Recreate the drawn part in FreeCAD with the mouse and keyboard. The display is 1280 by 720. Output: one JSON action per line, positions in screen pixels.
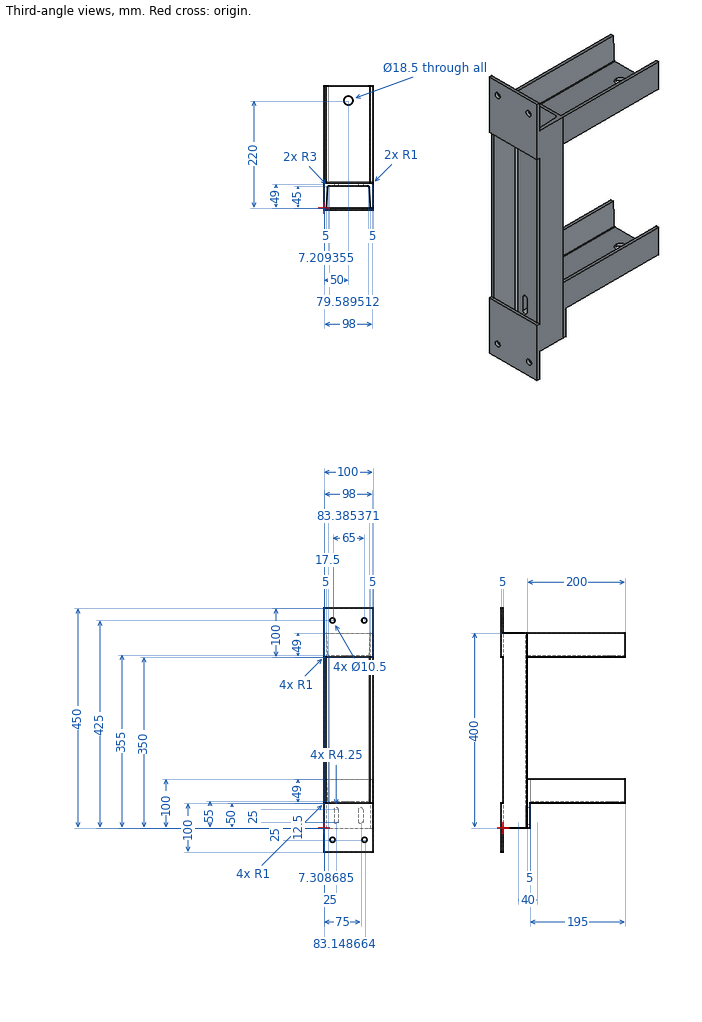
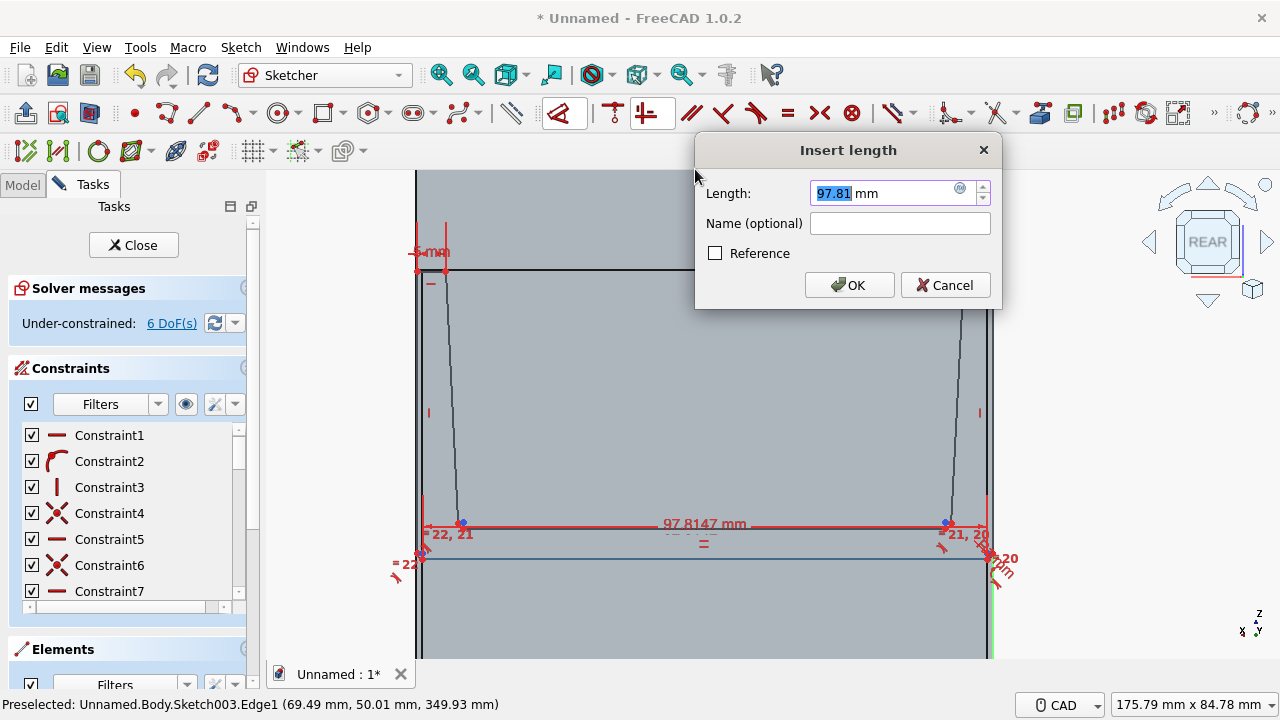
{"action": "type", "text": "98"}
{"action": "key", "text": "Return"}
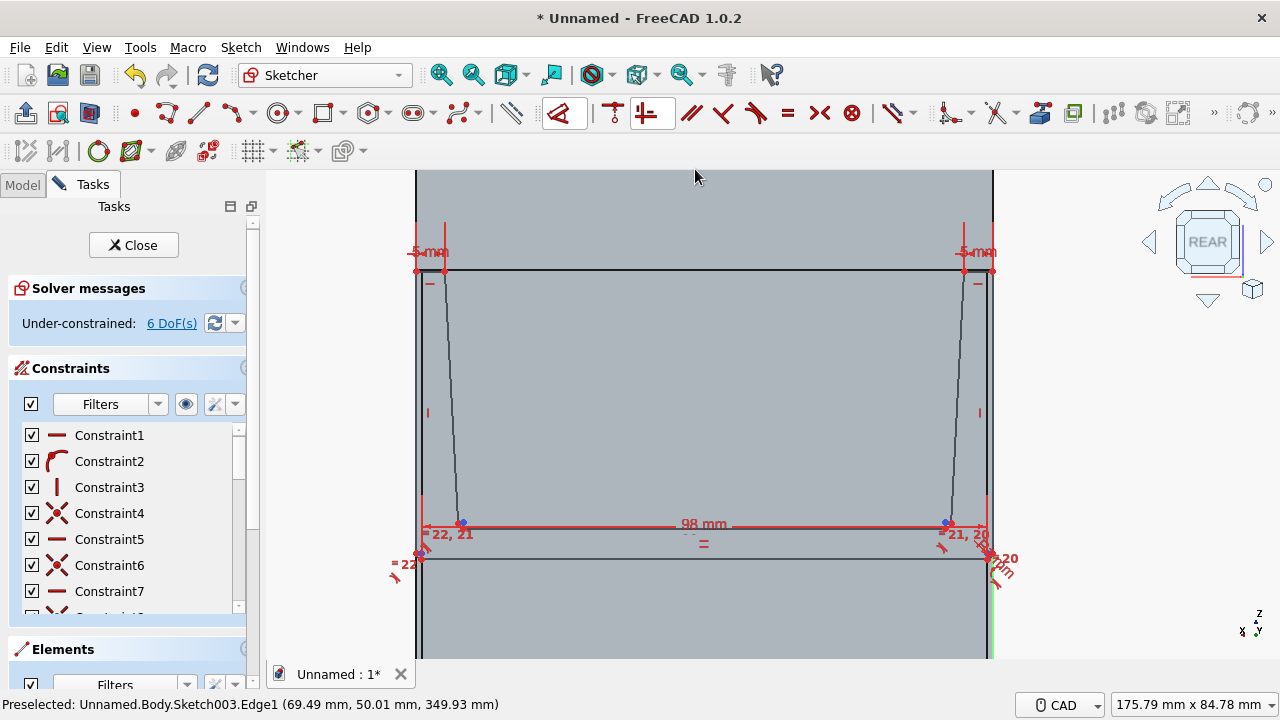
{"action": "left_click", "coordinate": [993, 469]}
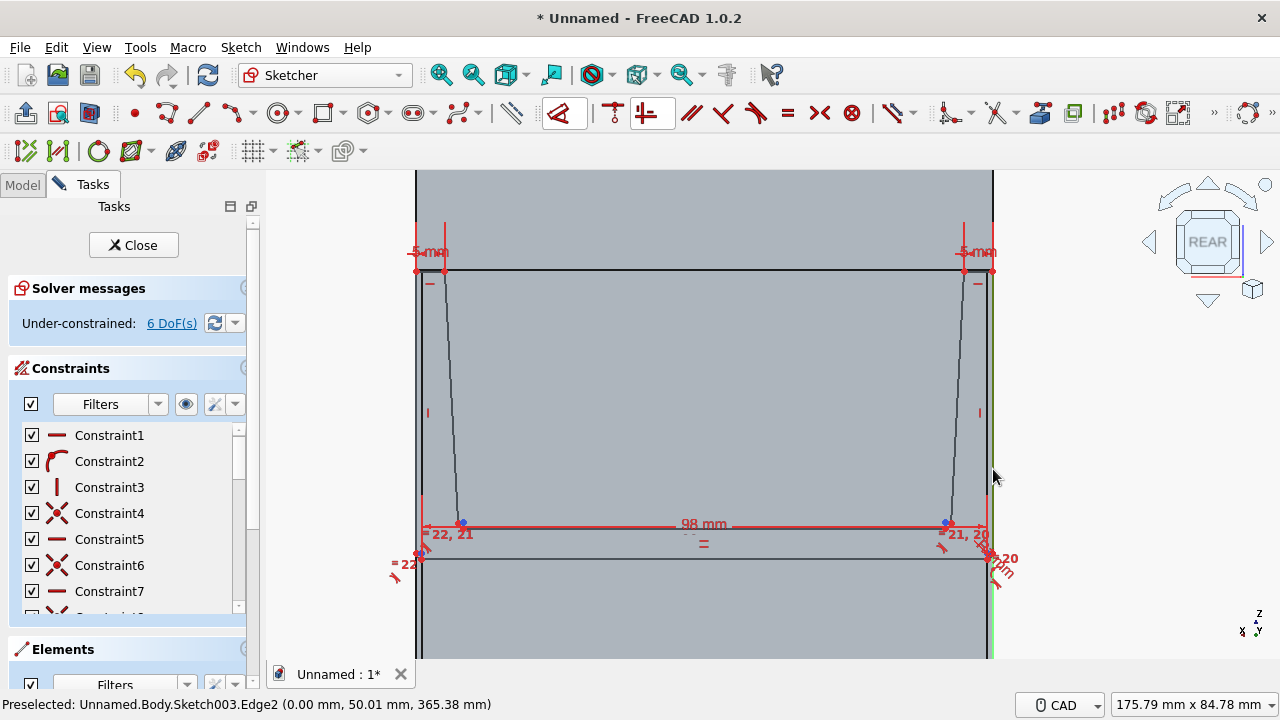
{"action": "key", "text": "i"}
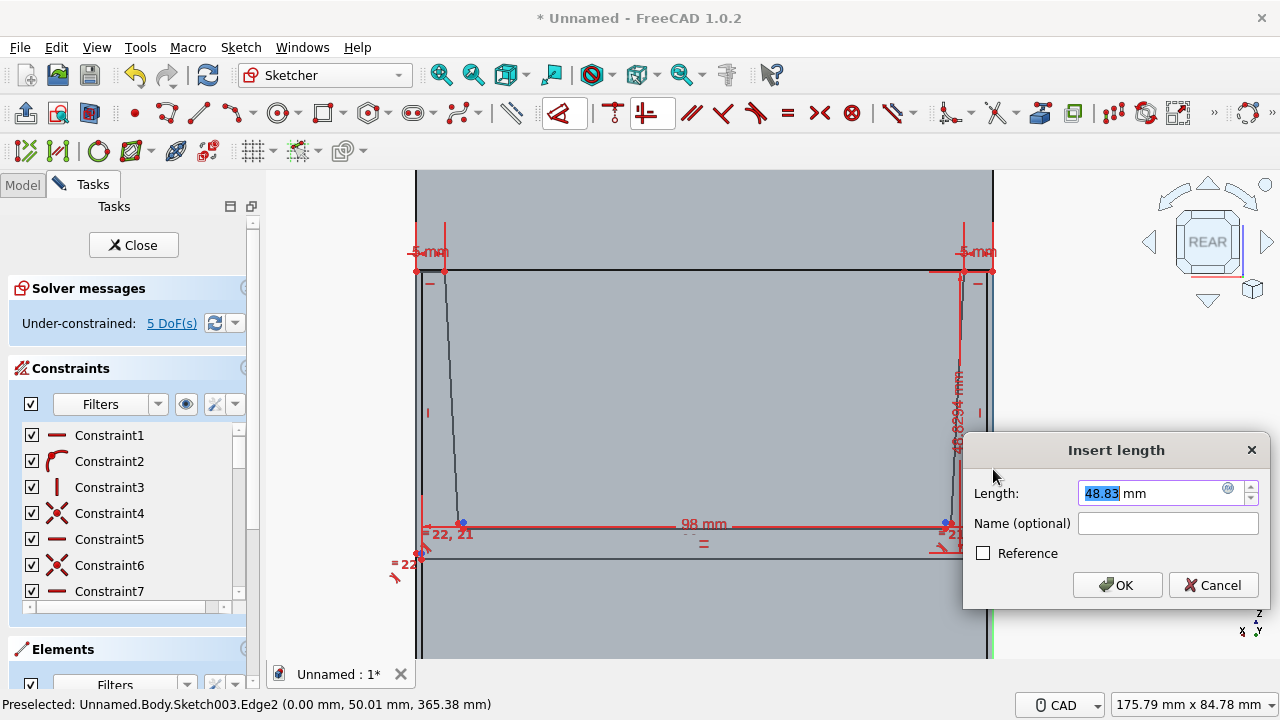
{"action": "type", "text": "49"}
{"action": "key", "text": "Return"}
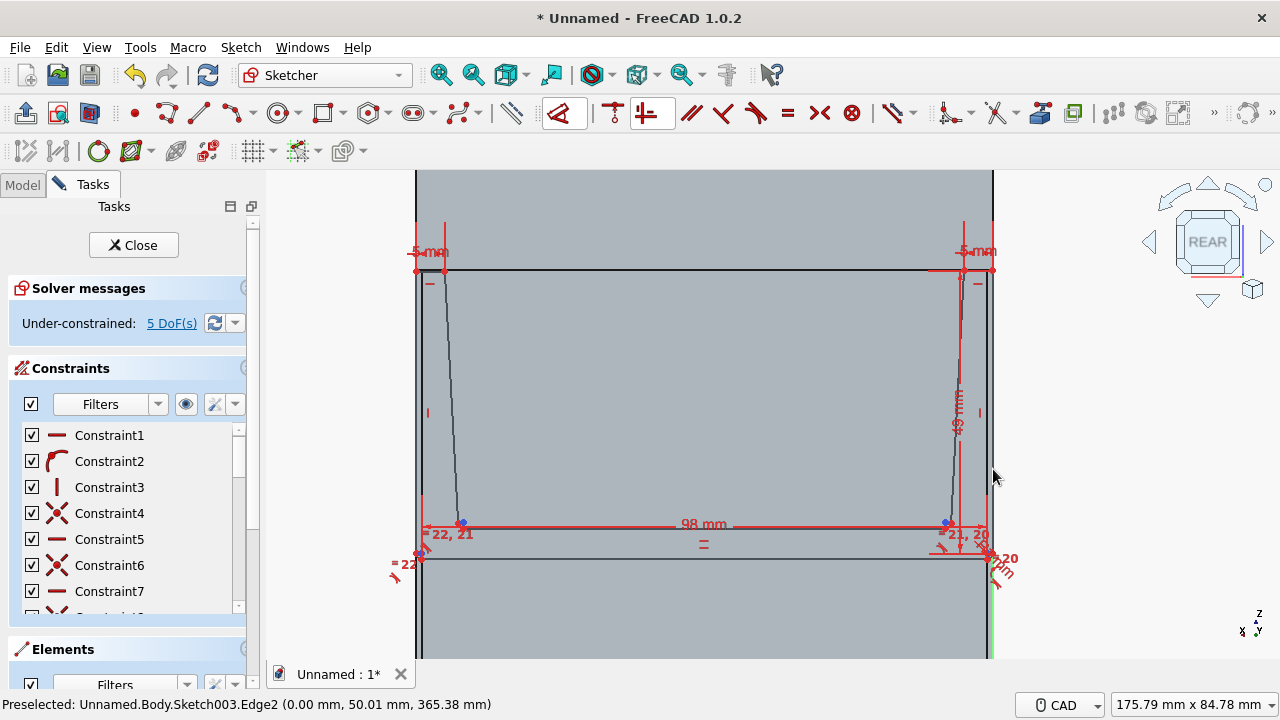
{"action": "left_click", "coordinate": [416, 356]}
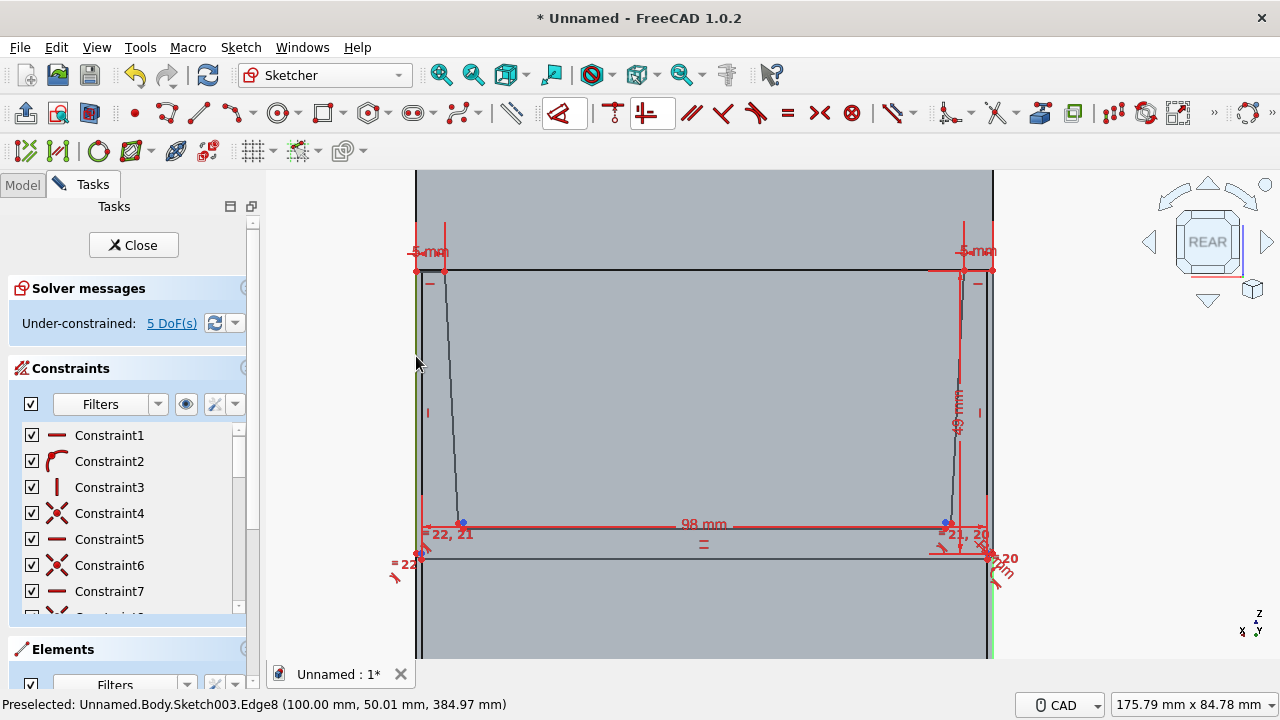
{"action": "left_click", "coordinate": [582, 114]}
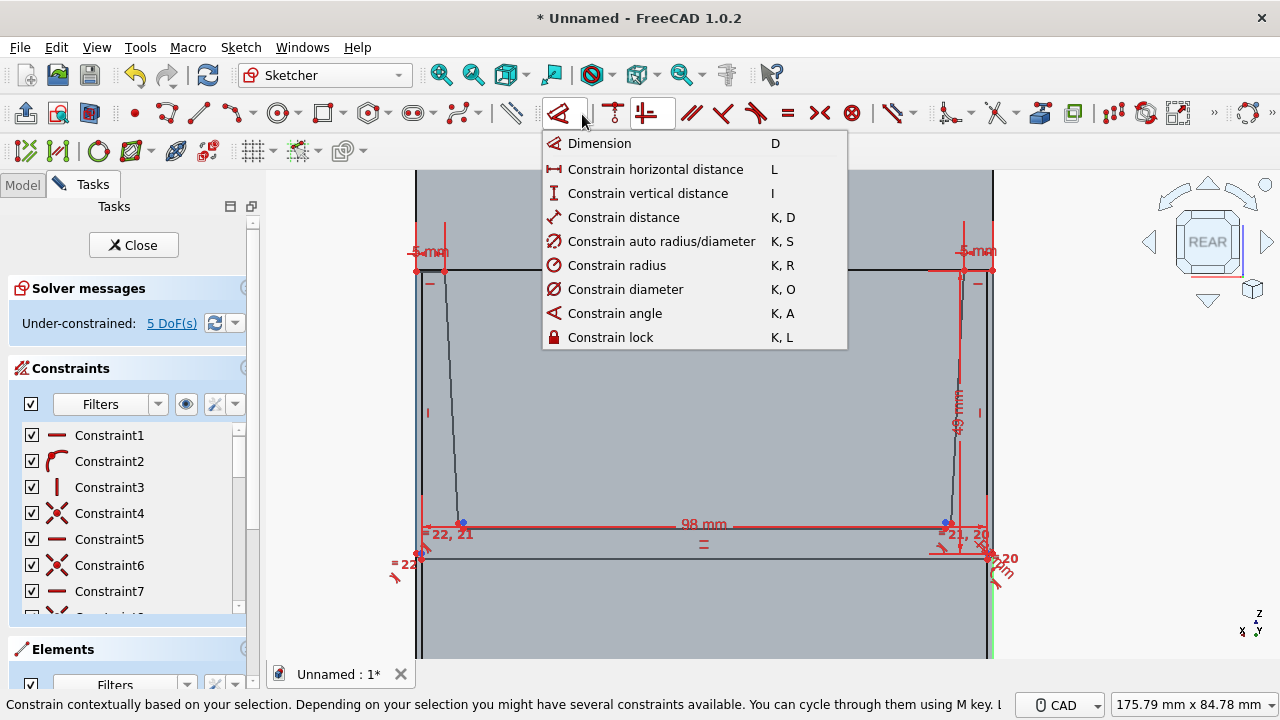
{"action": "left_click", "coordinate": [695, 193]}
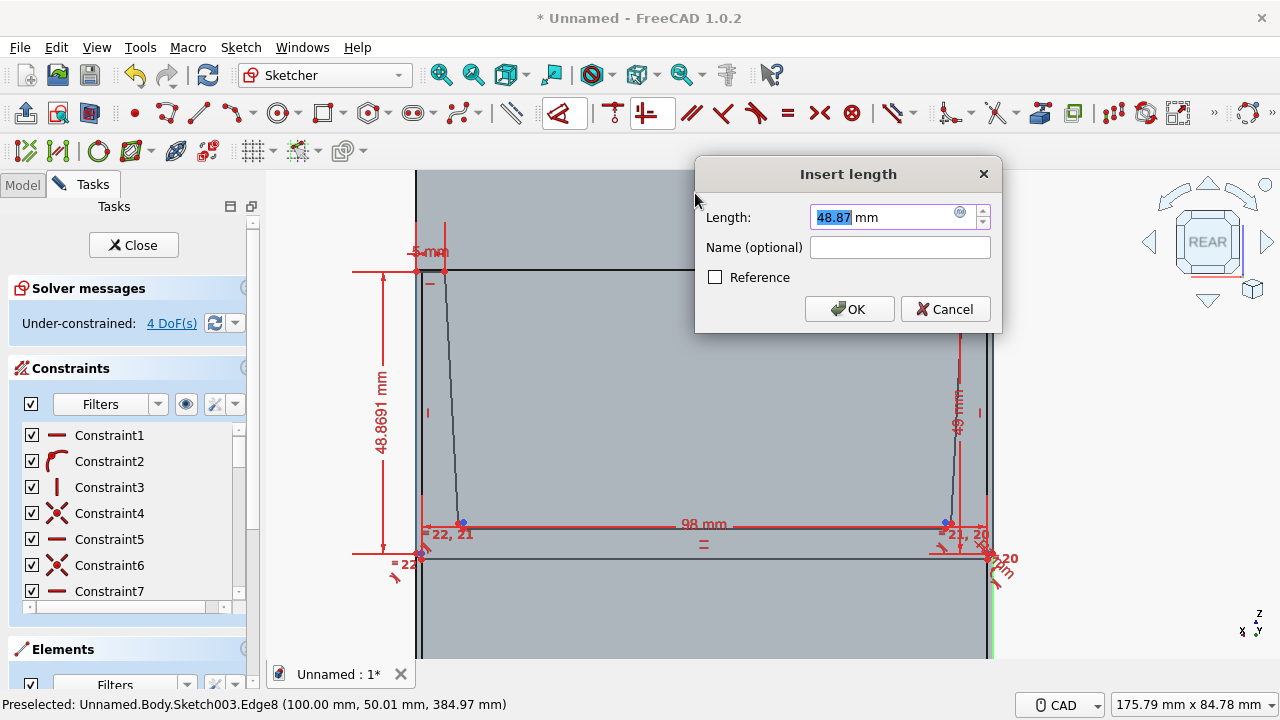
{"action": "type", "text": "49"}
{"action": "key", "text": "Return"}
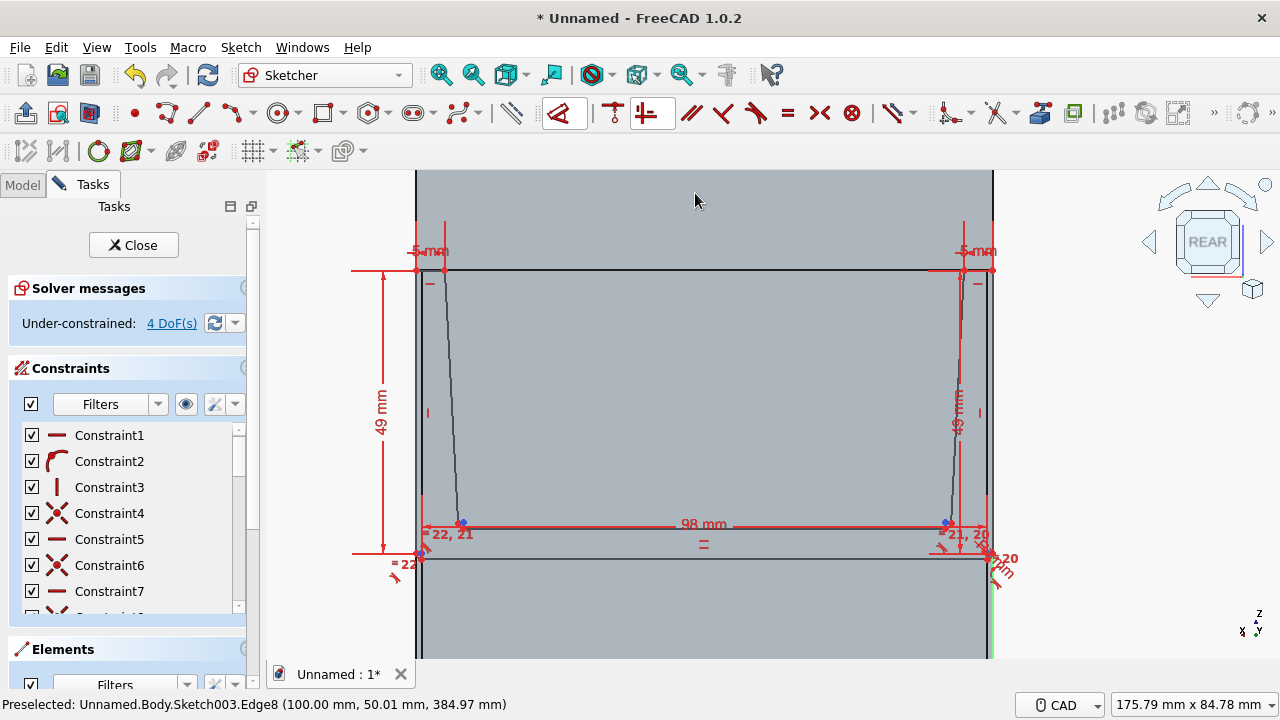
{"action": "scroll", "coordinate": [422, 559], "scroll_direction": "up", "scroll_amount": 4}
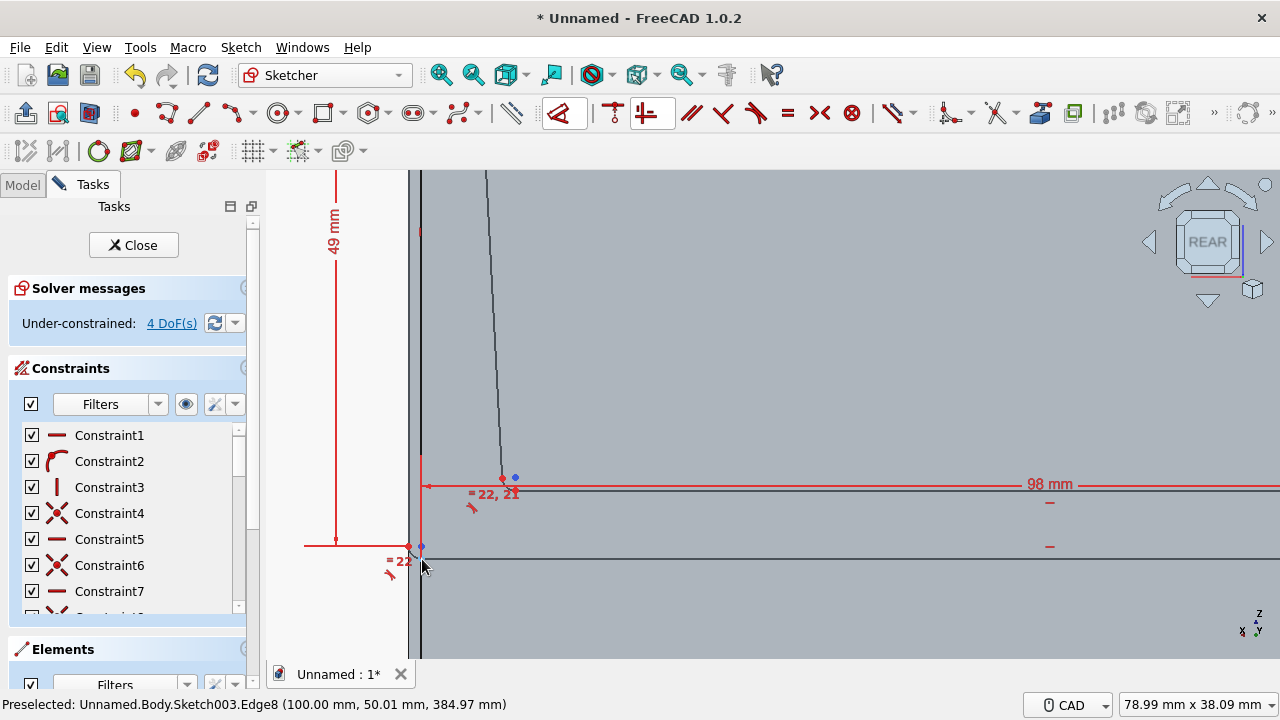
{"action": "left_click", "coordinate": [421, 559]}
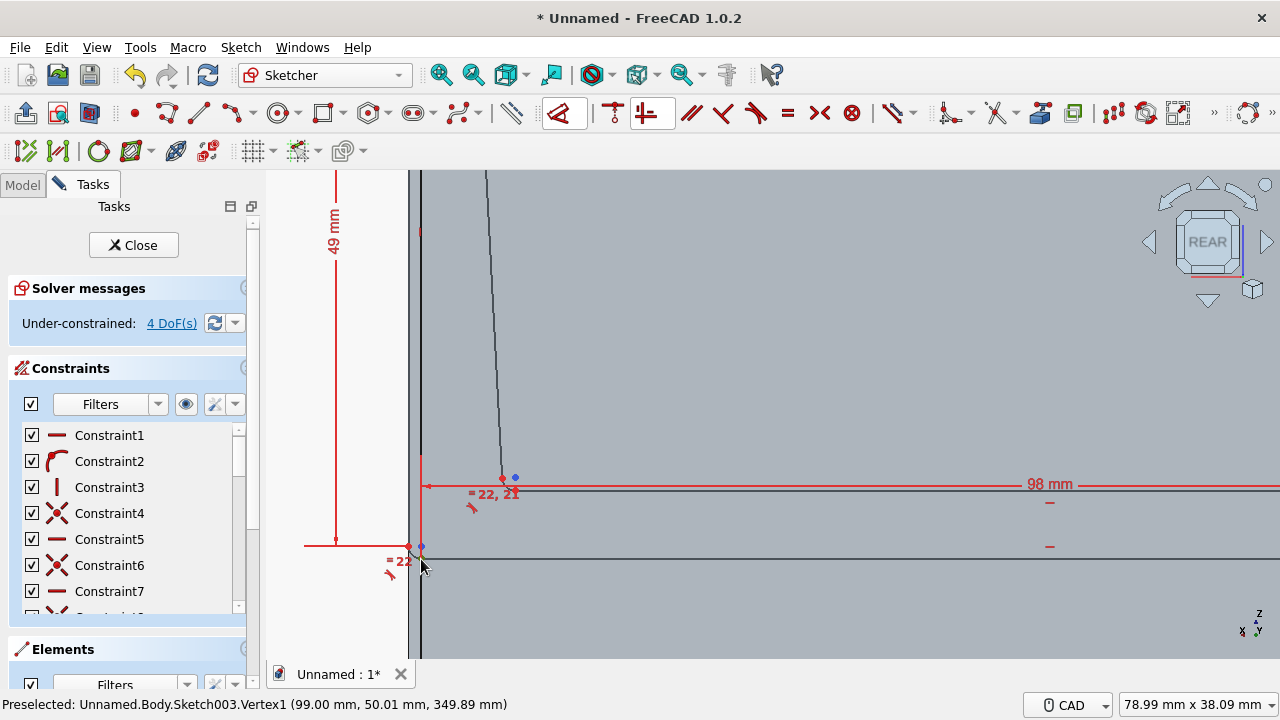
{"action": "left_click", "coordinate": [582, 114]}